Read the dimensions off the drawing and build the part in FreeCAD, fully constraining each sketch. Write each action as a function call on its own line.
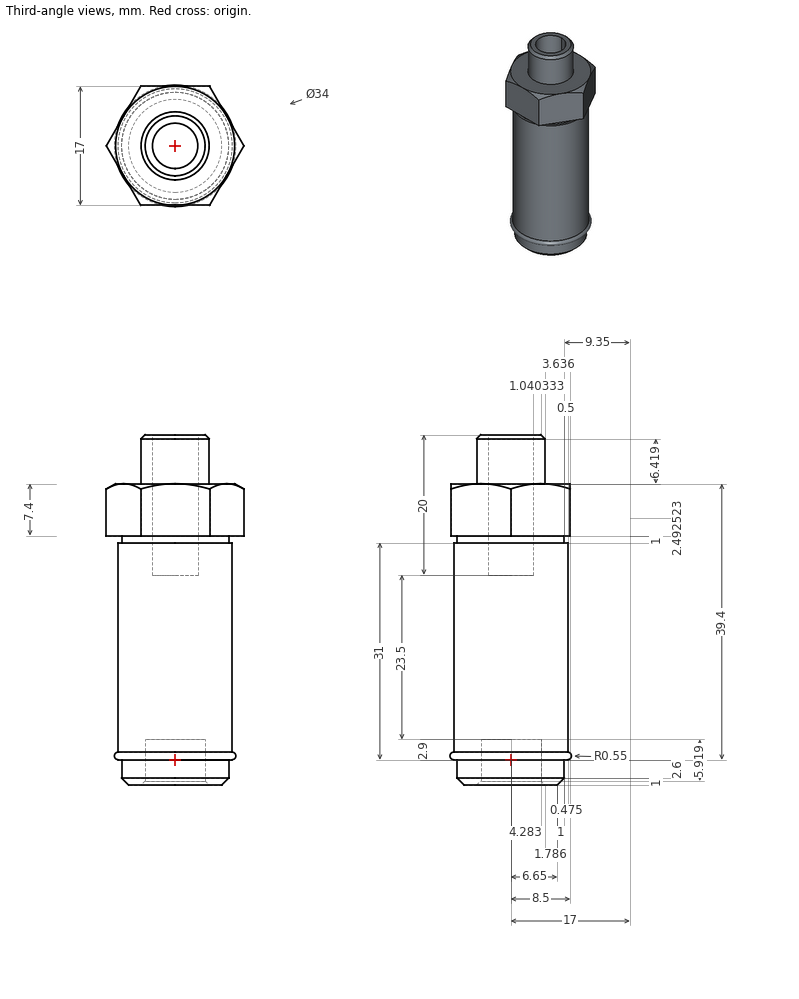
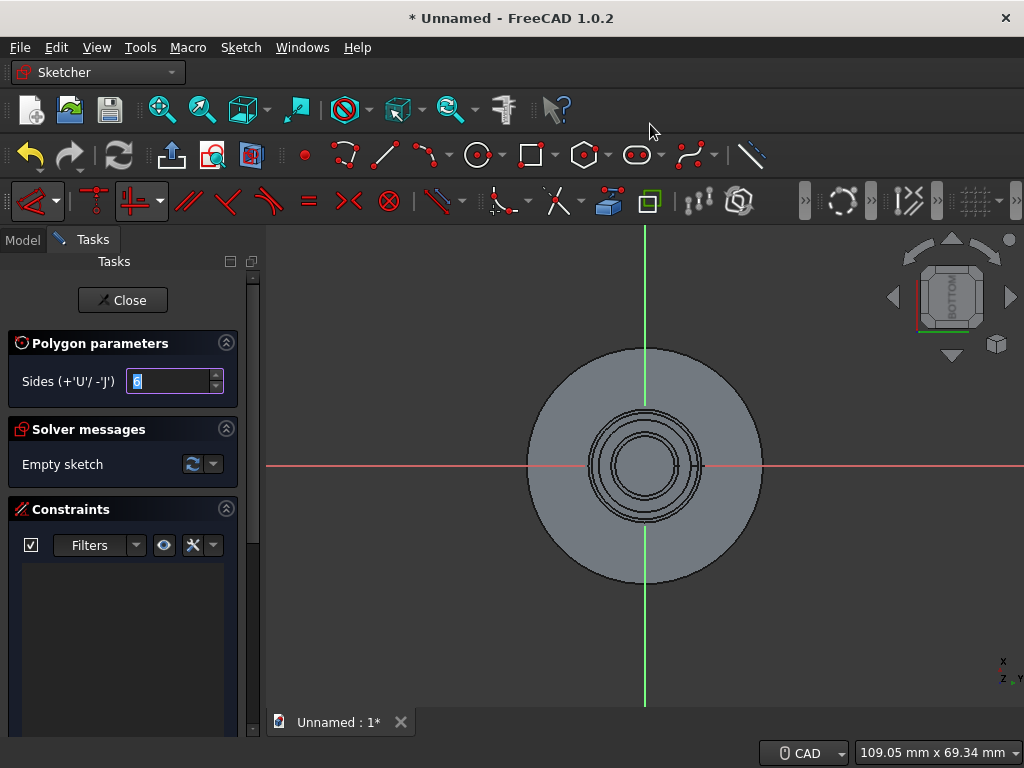
click(645, 466)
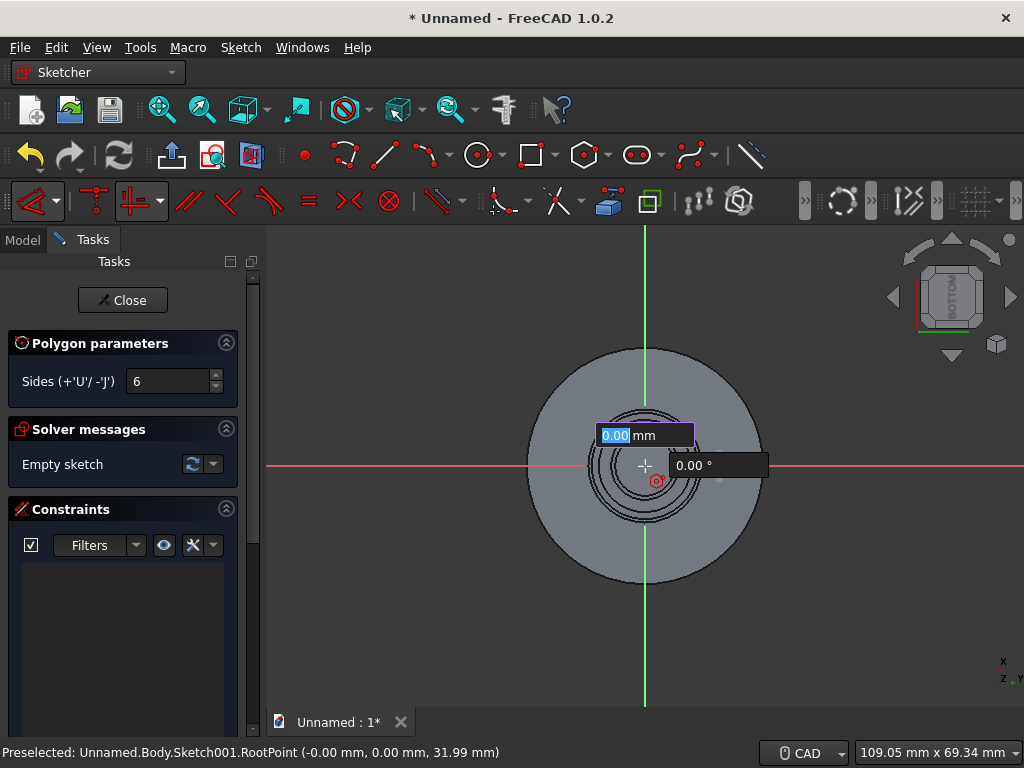
click(645, 534)
key(Escape)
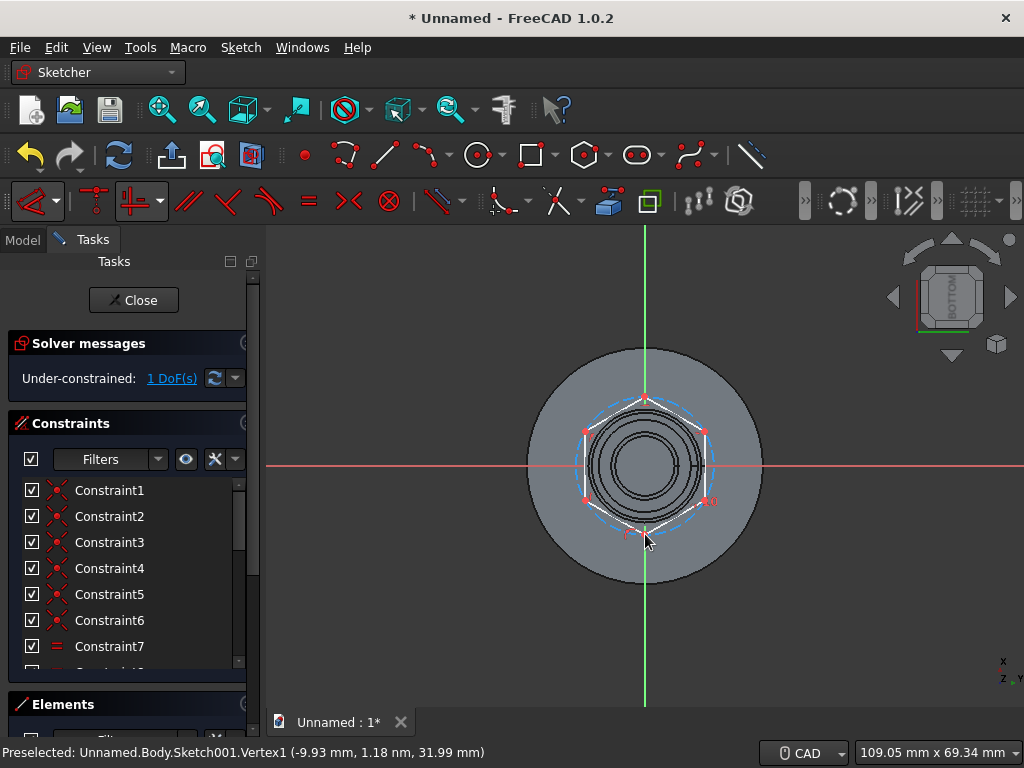
click(478, 156)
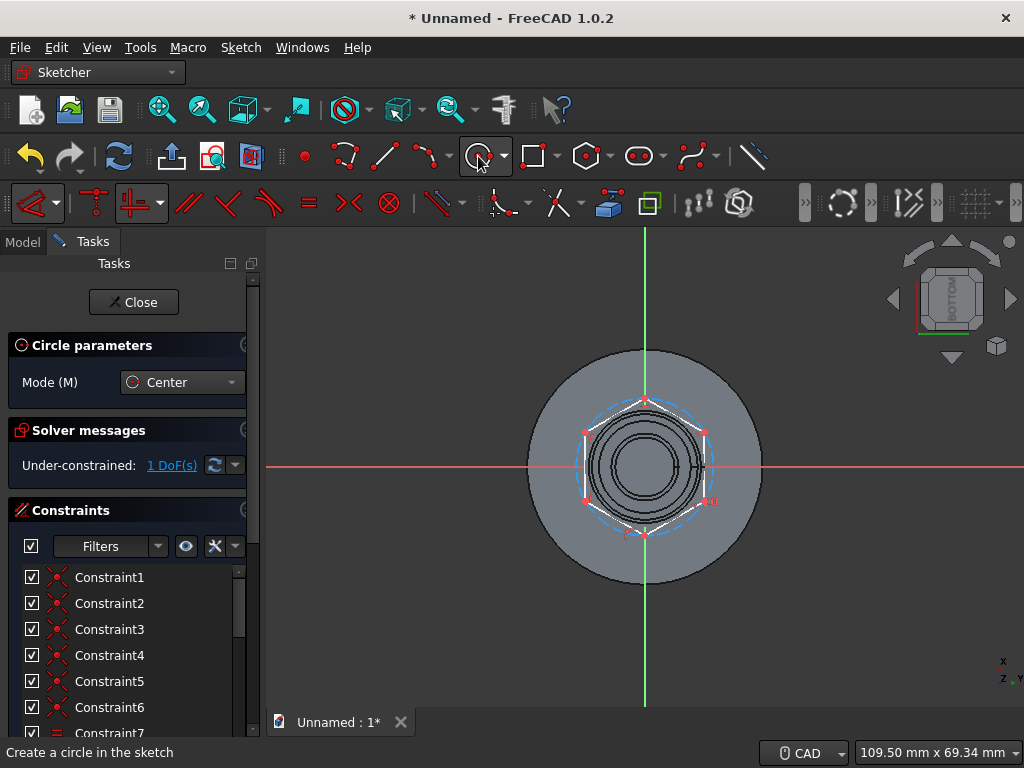
click(645, 467)
move(728, 384)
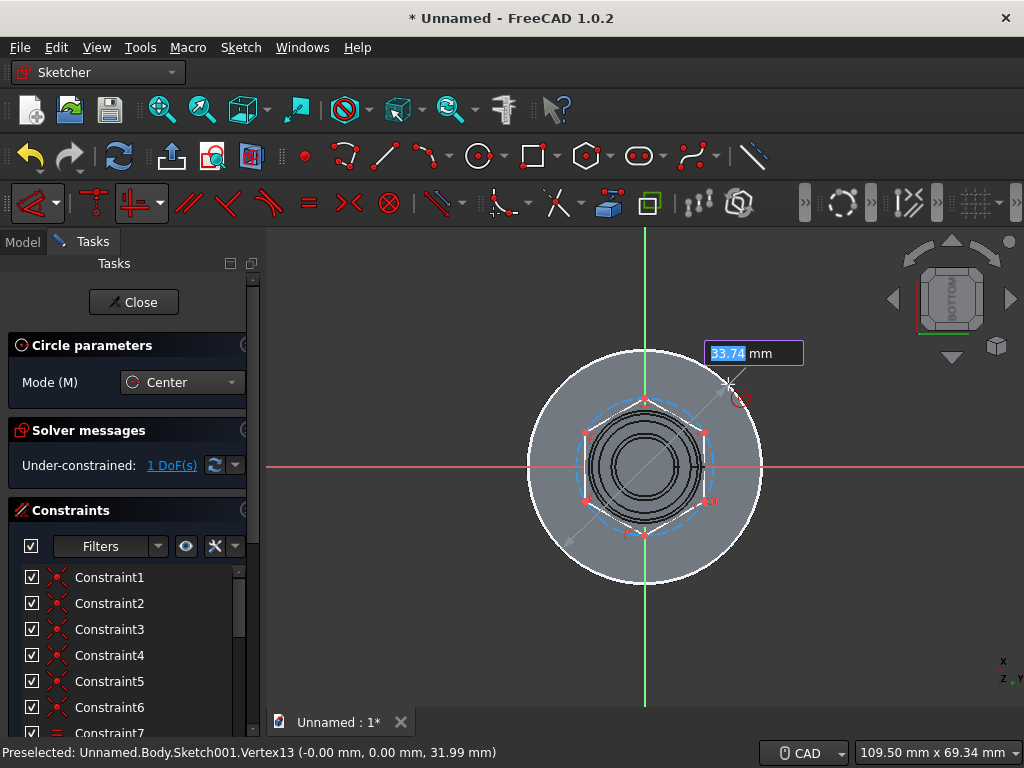
text(34)
key(Return)
key(Escape)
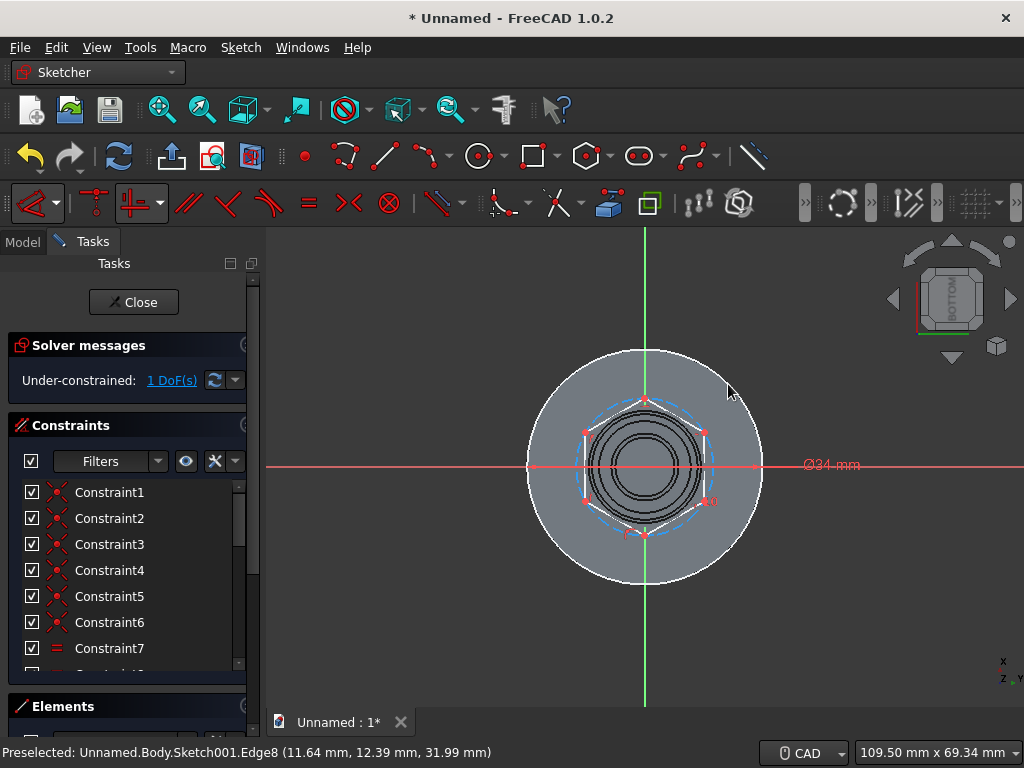
click(585, 433)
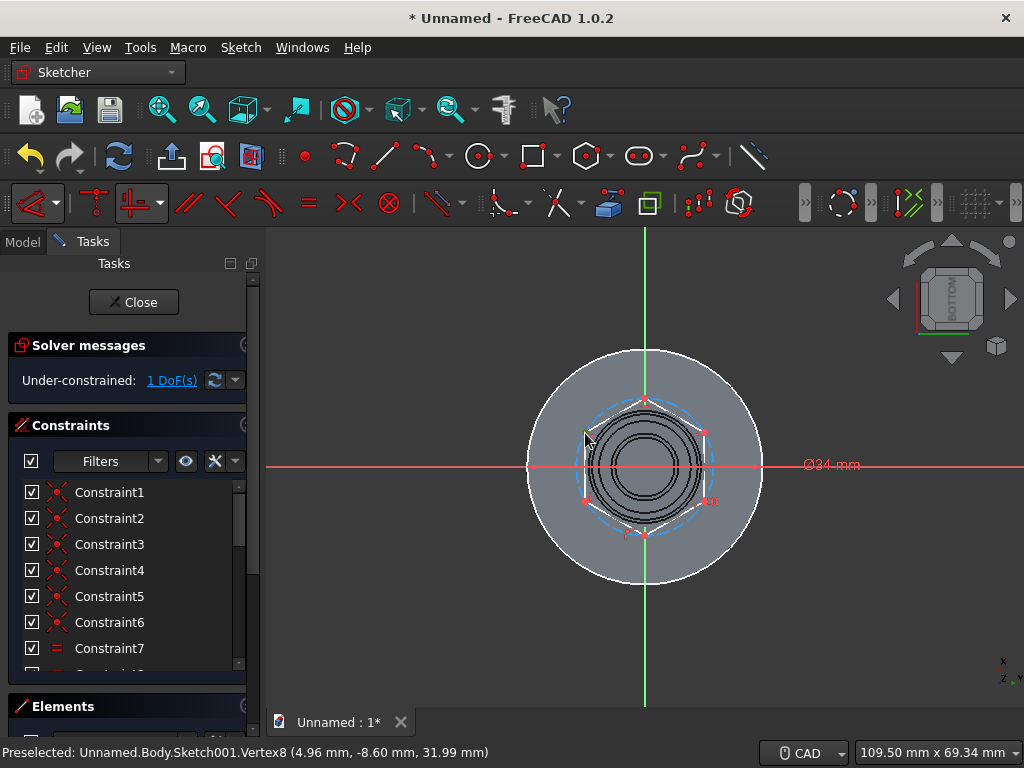
click(704, 501)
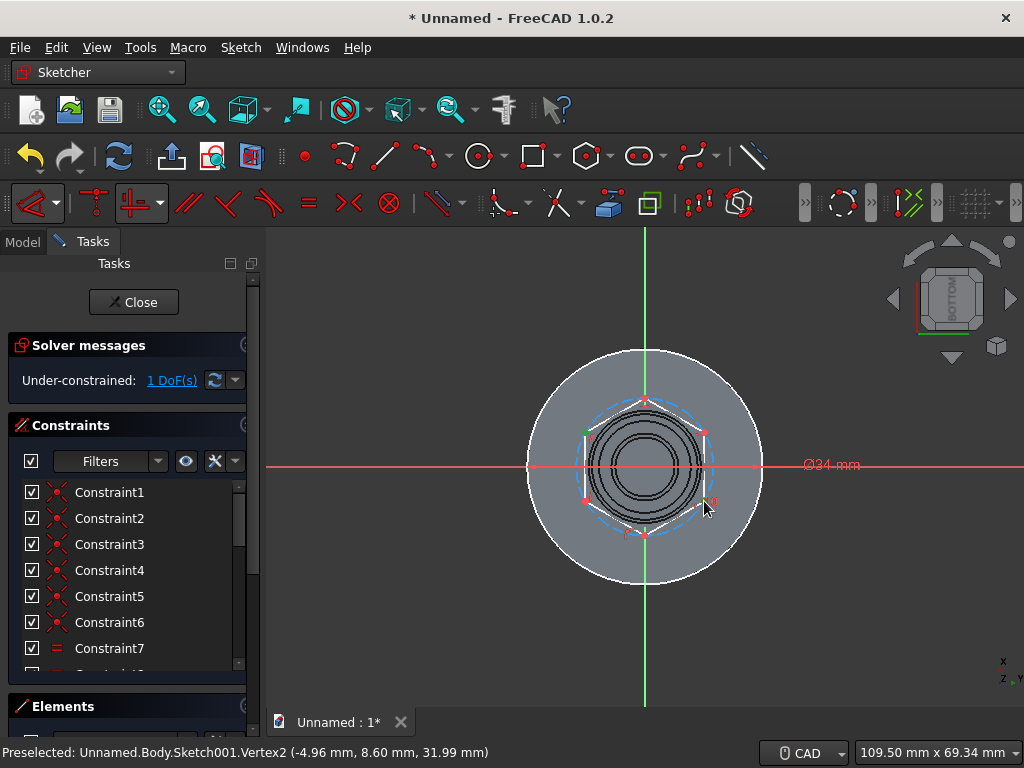
key(l)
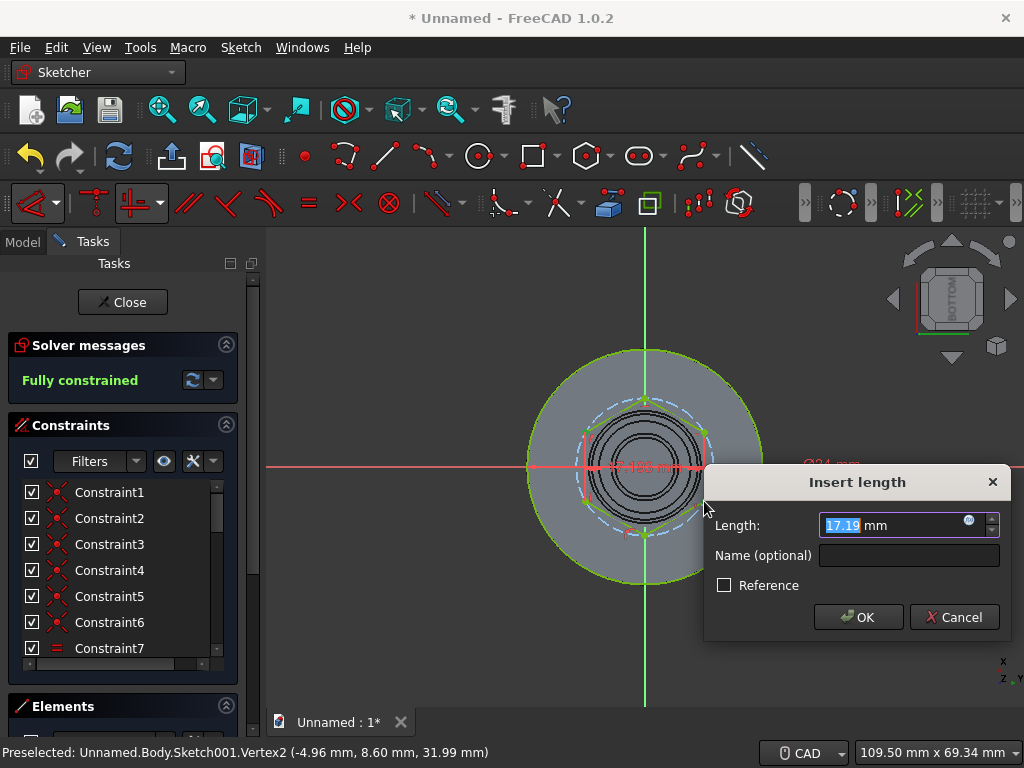
text(17)
key(Return)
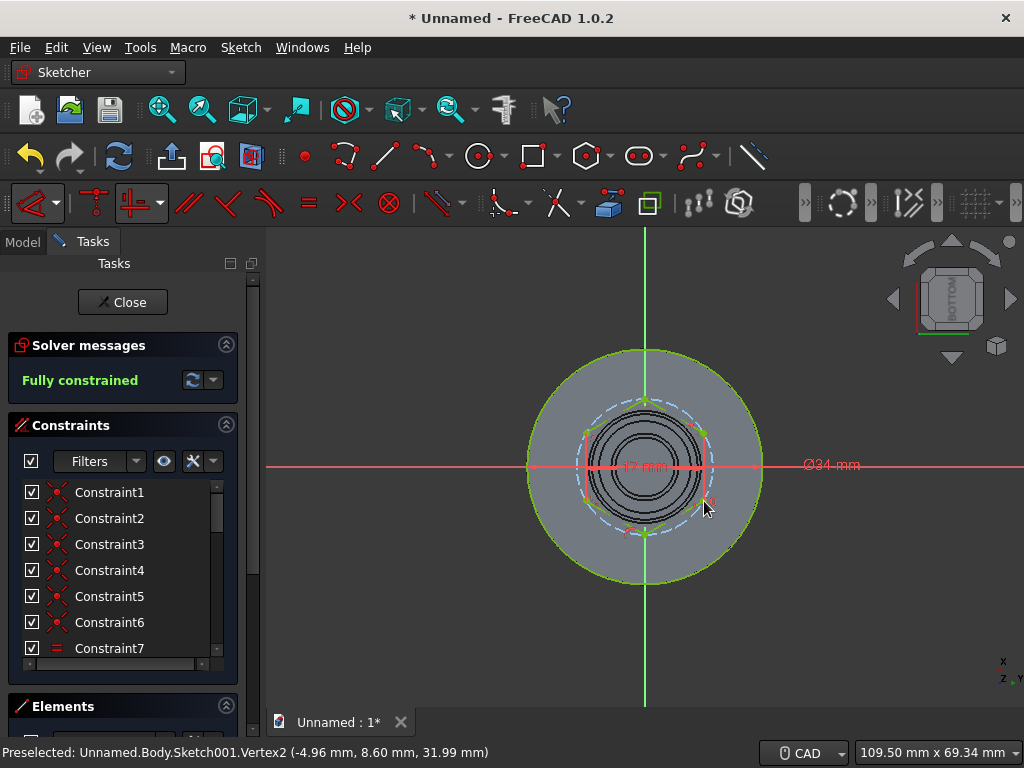
click(123, 302)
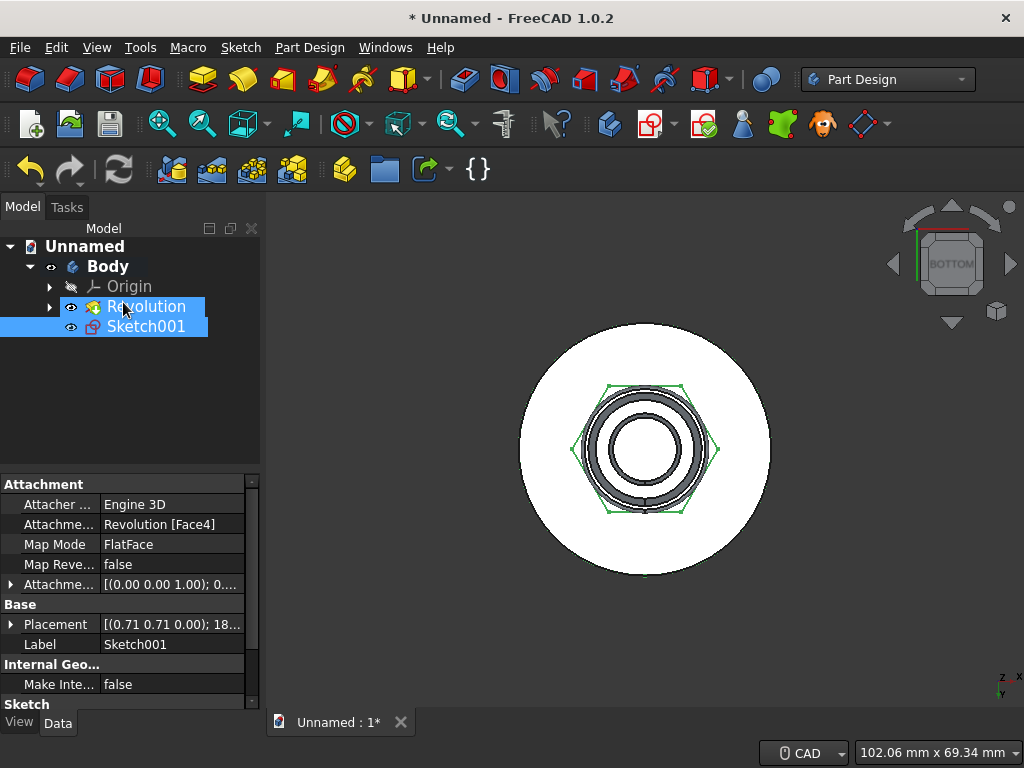
click(466, 80)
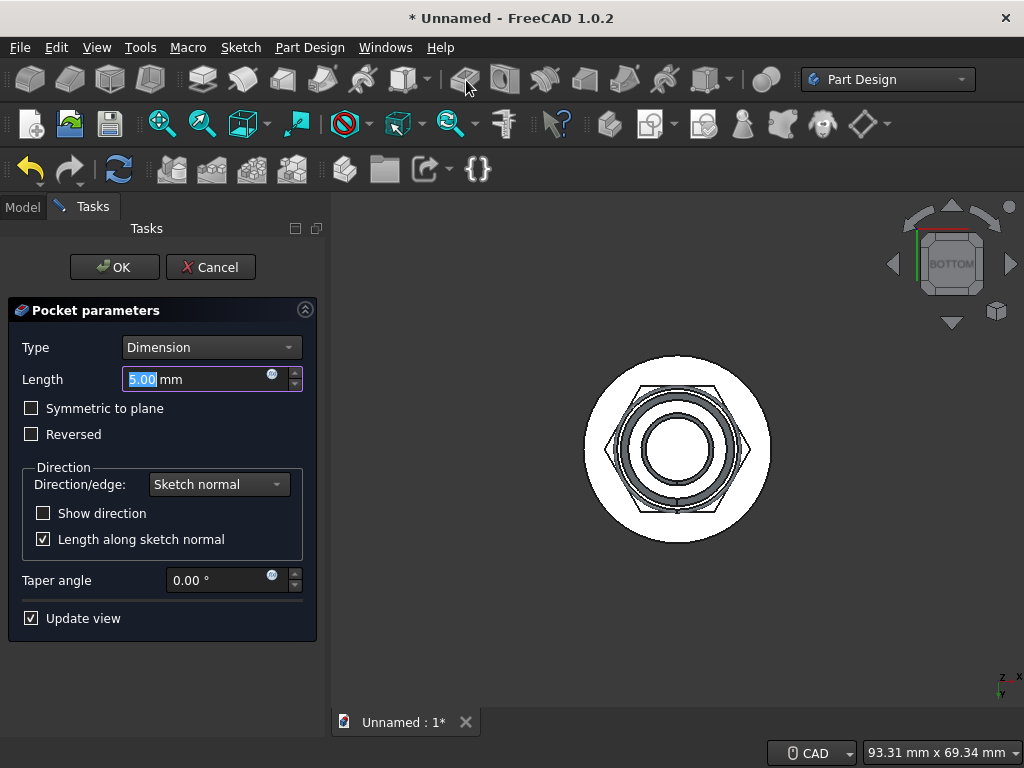
text(7.4)
key(Tab)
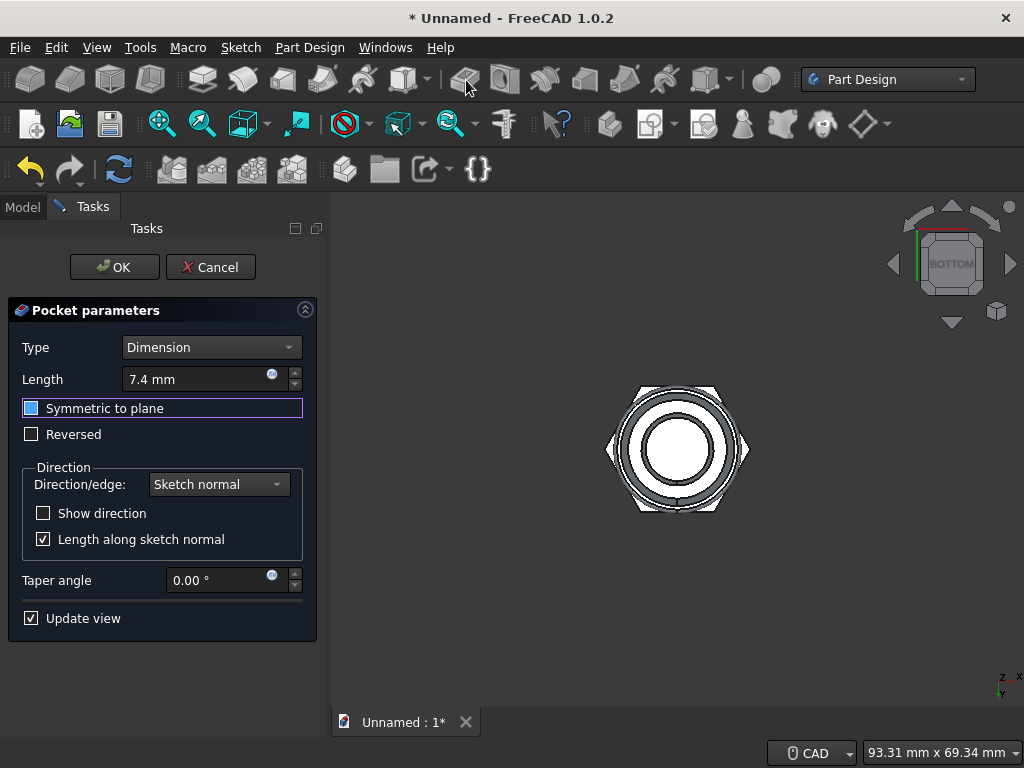
click(115, 267)